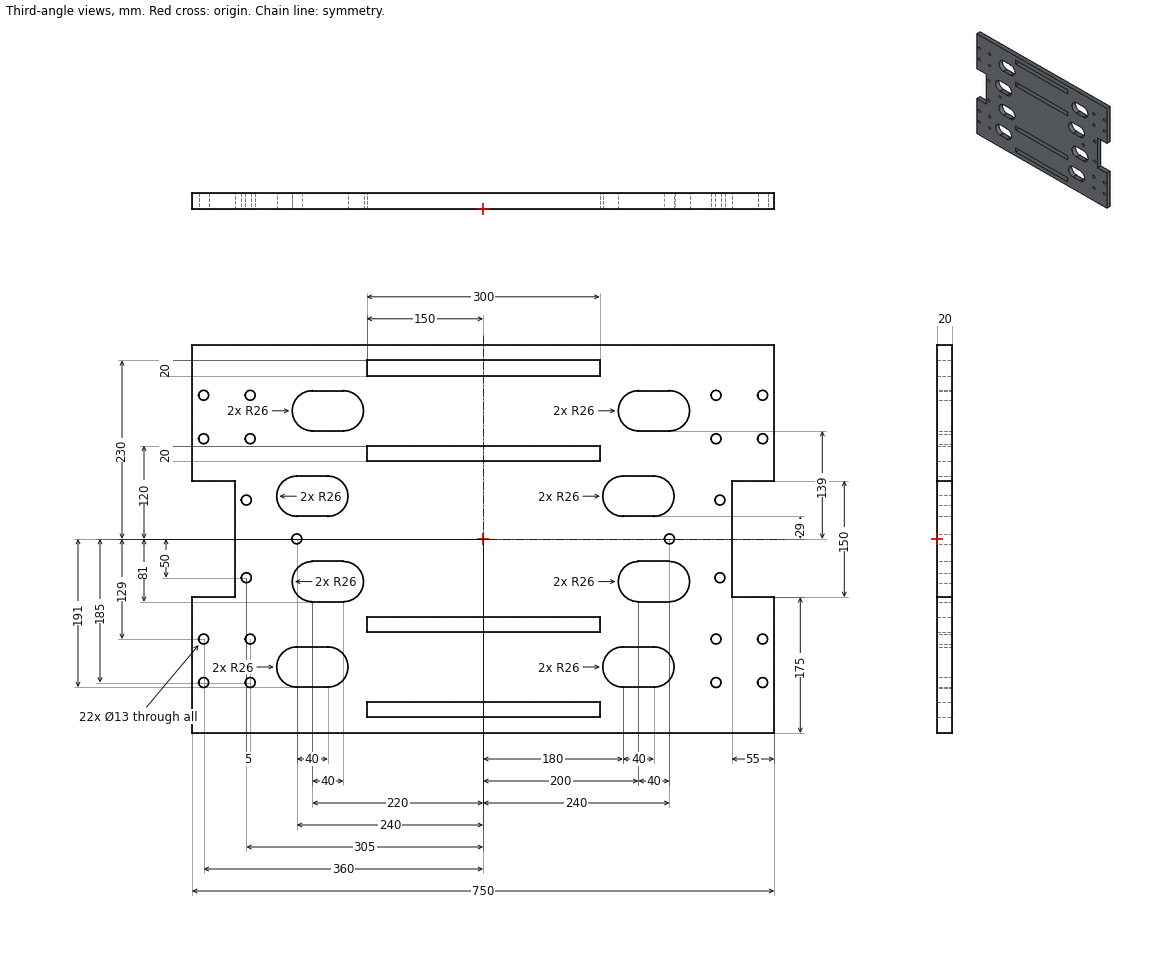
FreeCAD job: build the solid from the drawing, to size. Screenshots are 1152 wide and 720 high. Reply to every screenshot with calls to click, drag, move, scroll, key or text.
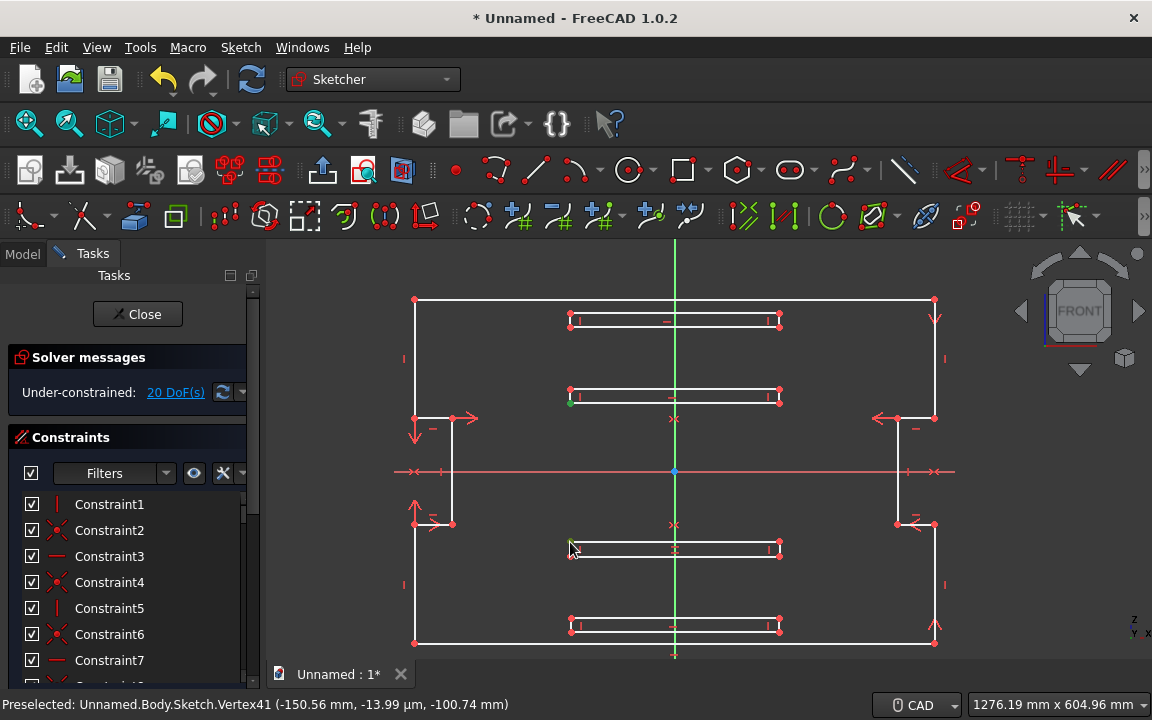
click(393, 472)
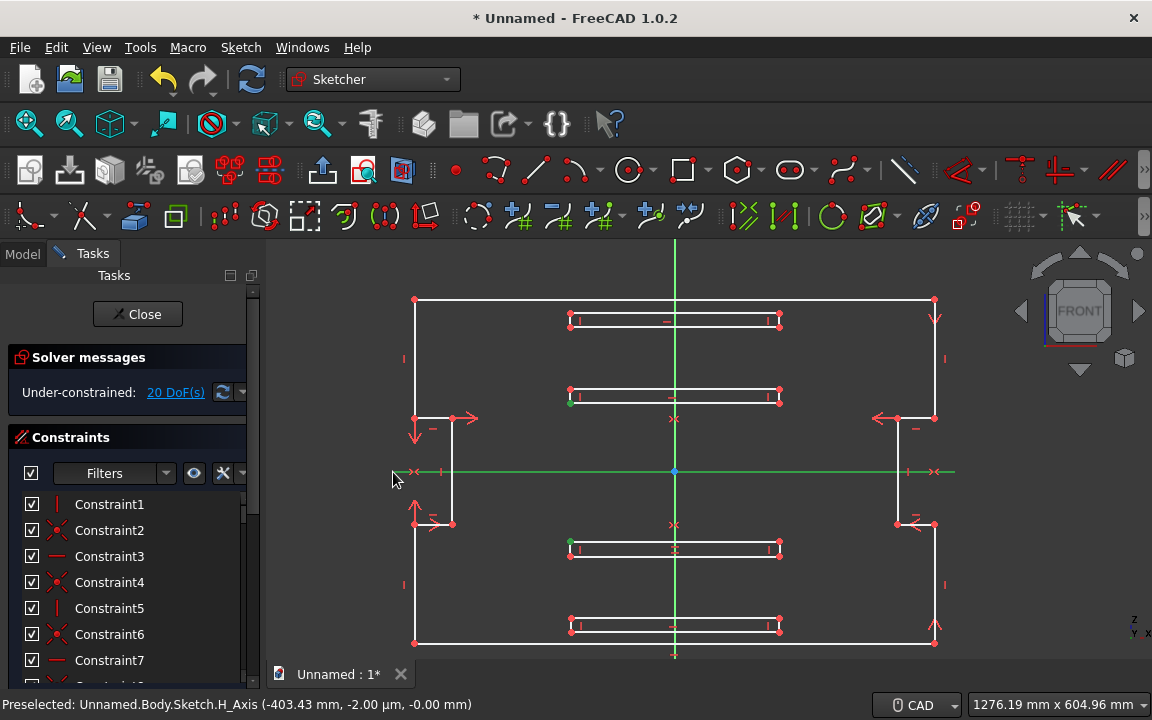
key(s)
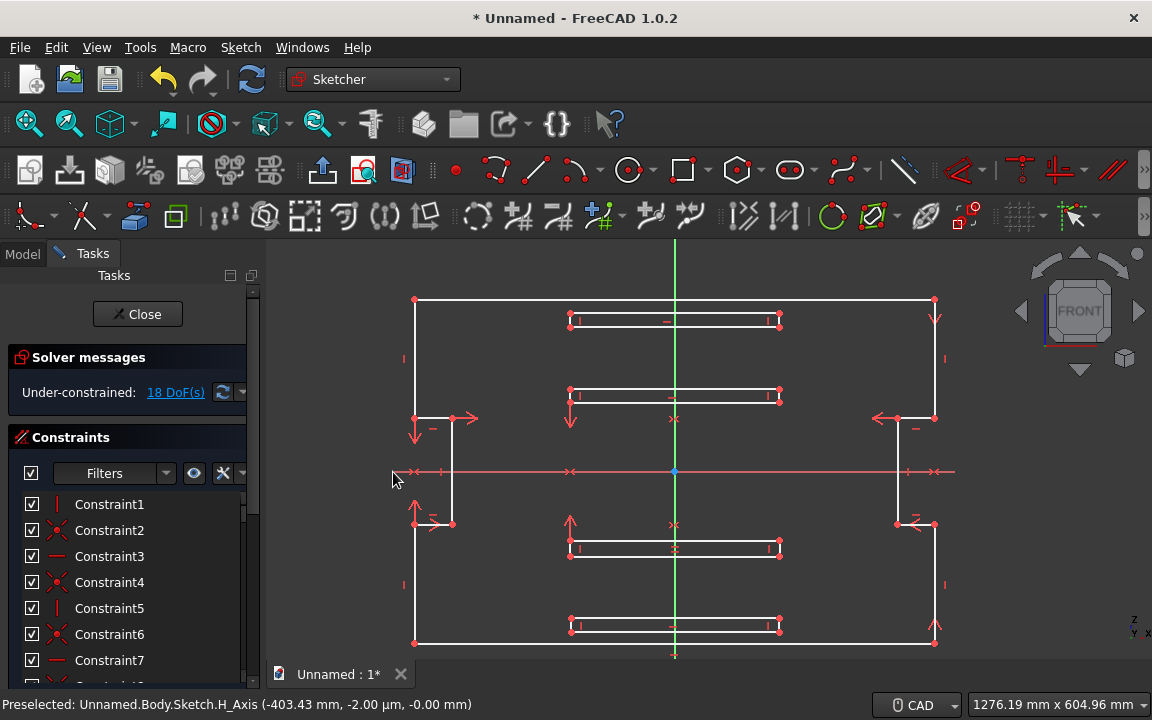
click(779, 389)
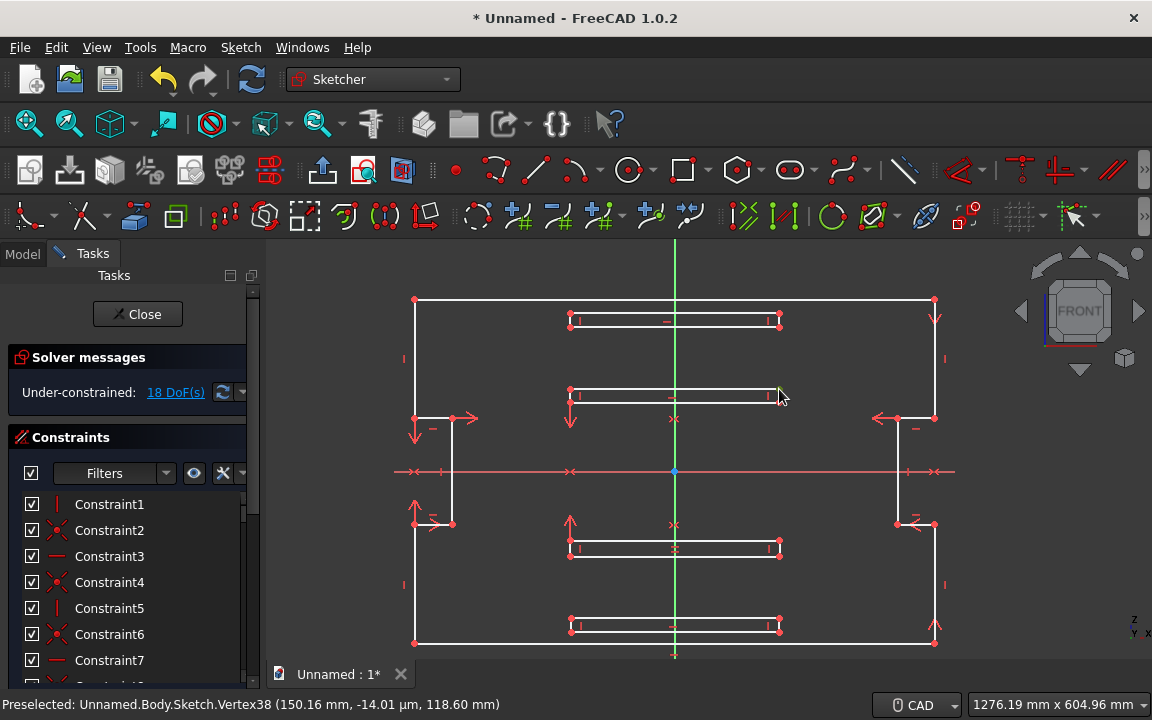
click(780, 557)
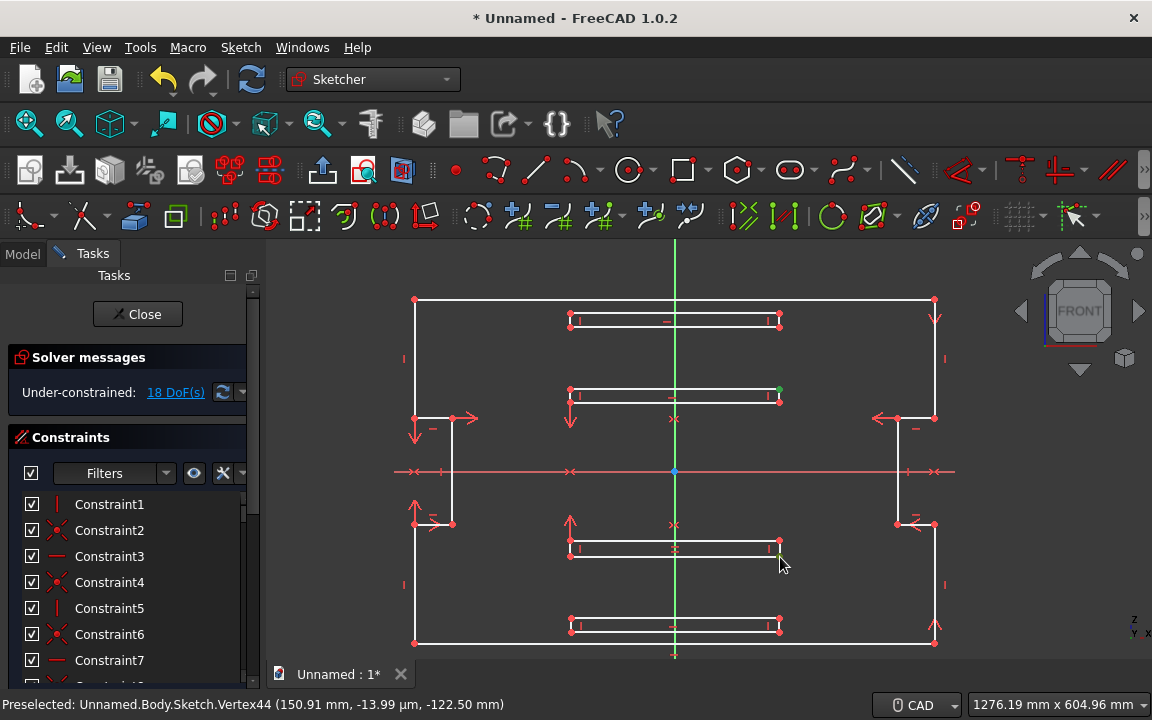
click(393, 472)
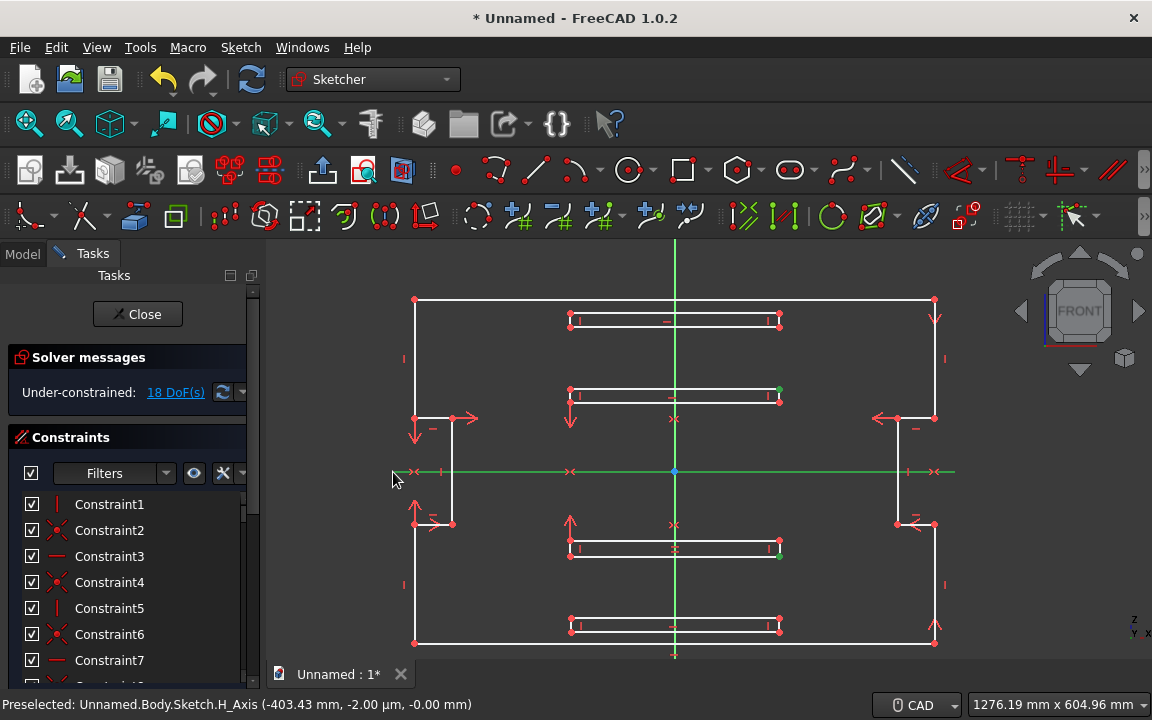
key(s)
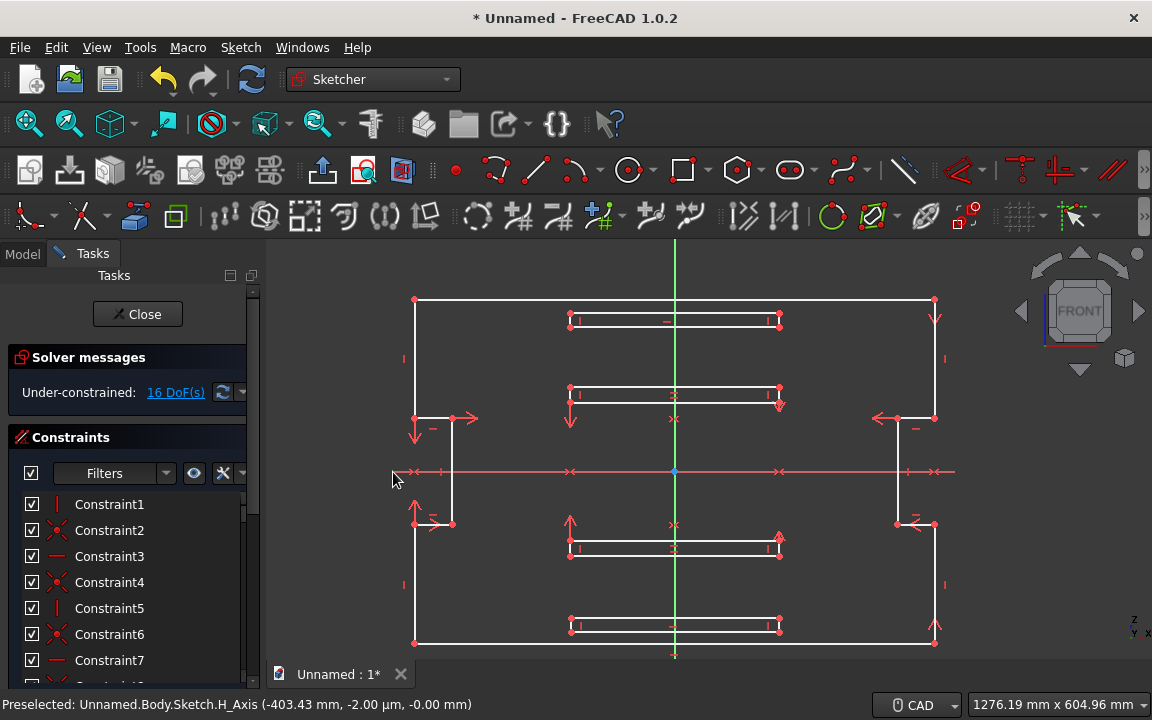
click(570, 327)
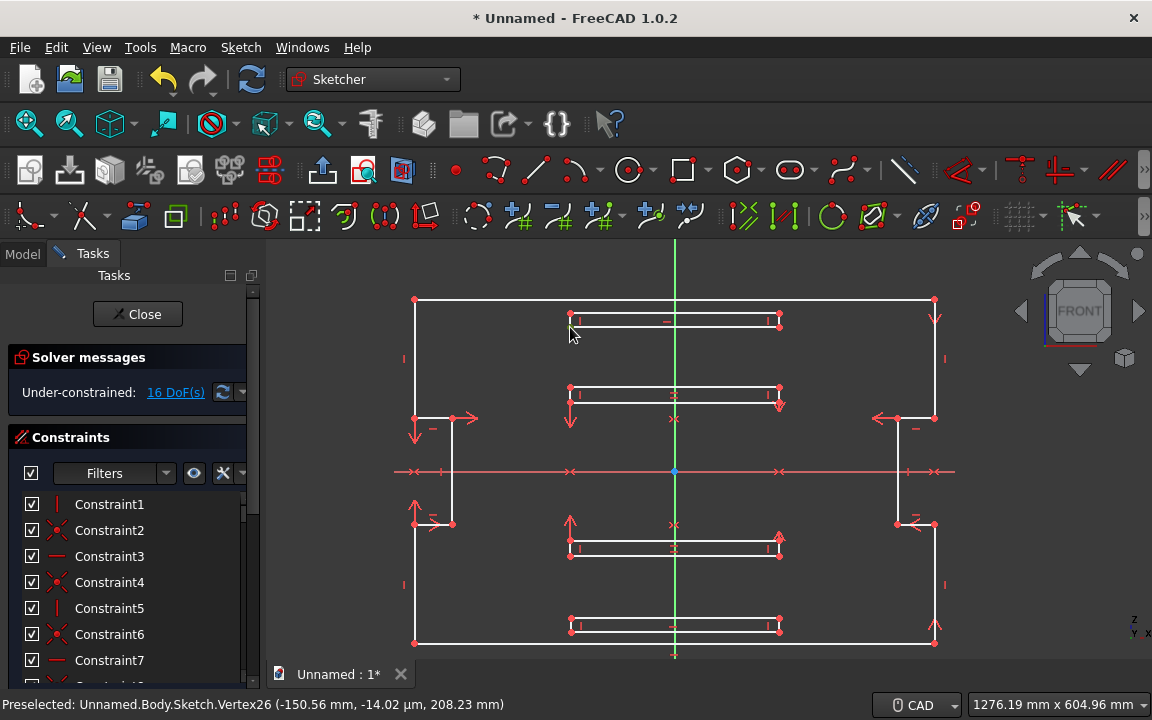
click(571, 618)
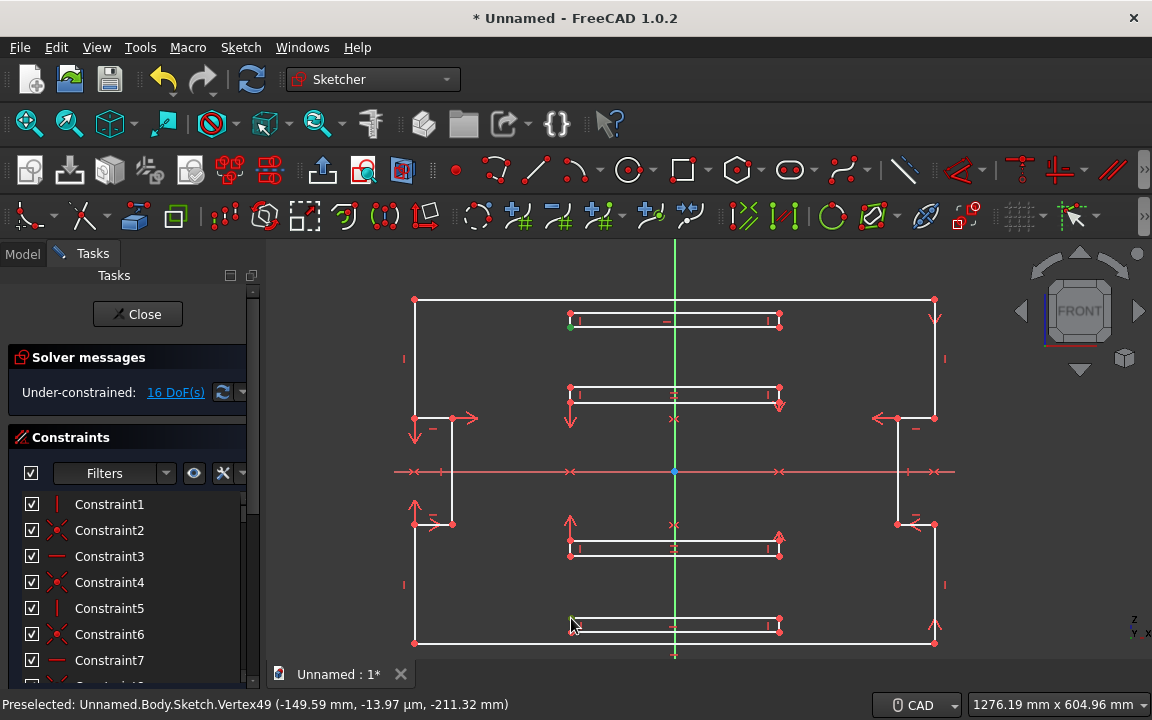
click(393, 472)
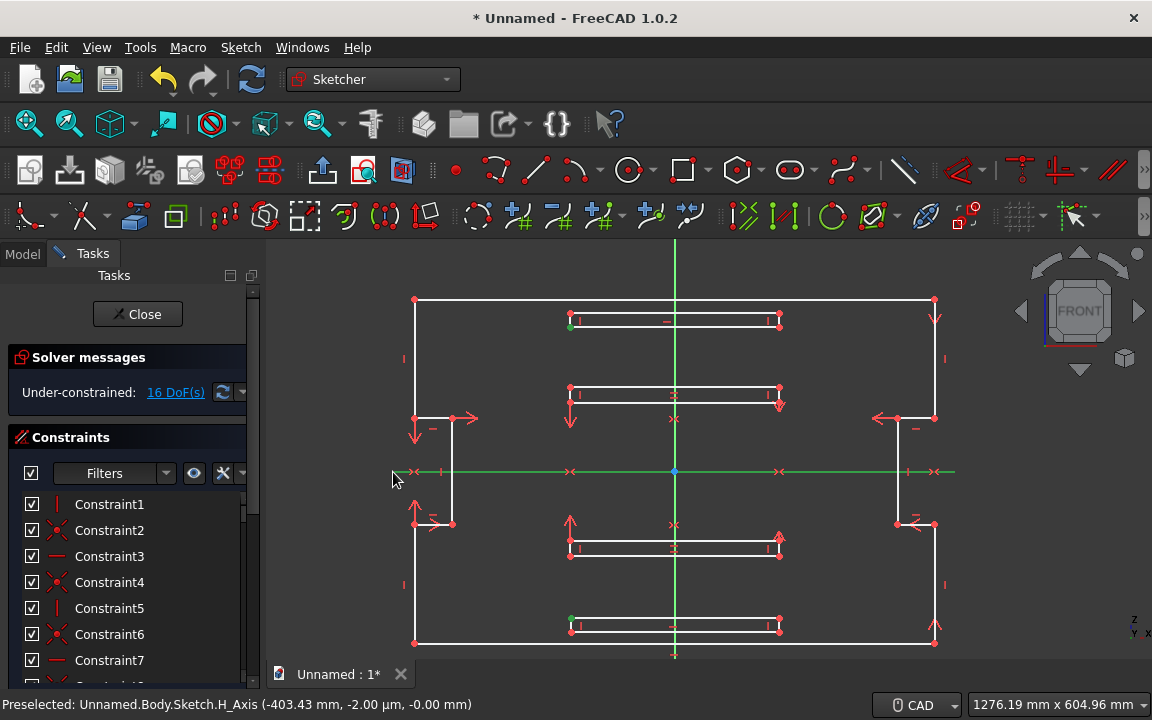
key(s)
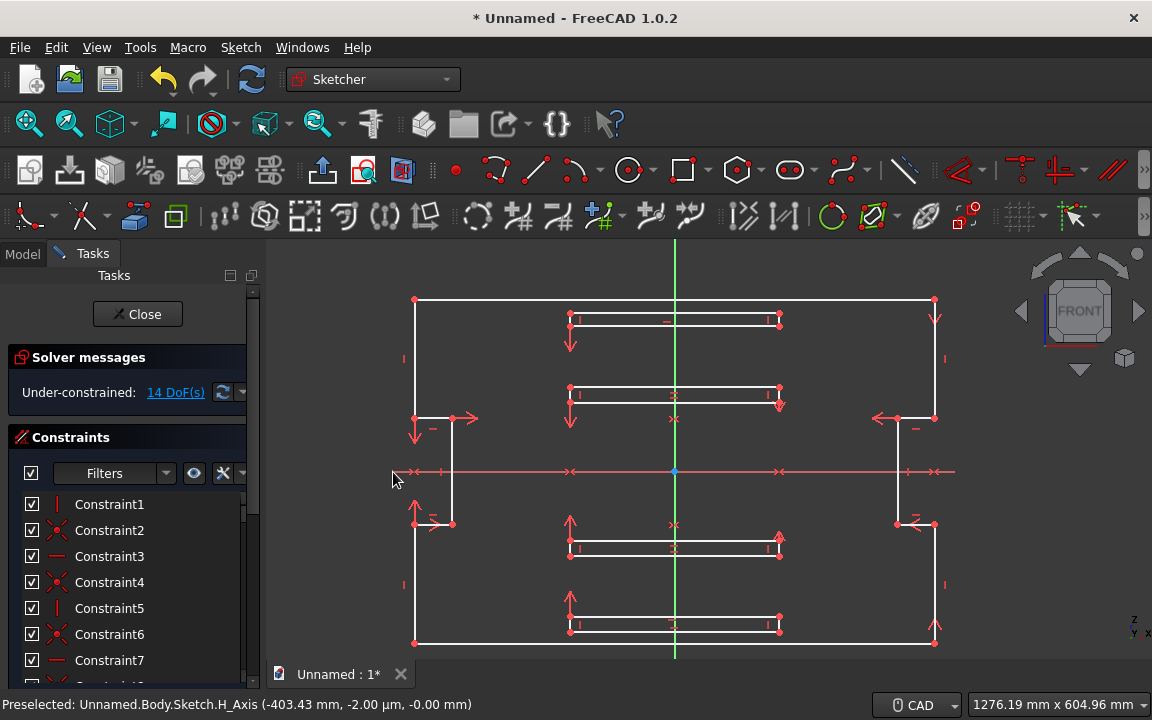
click(779, 313)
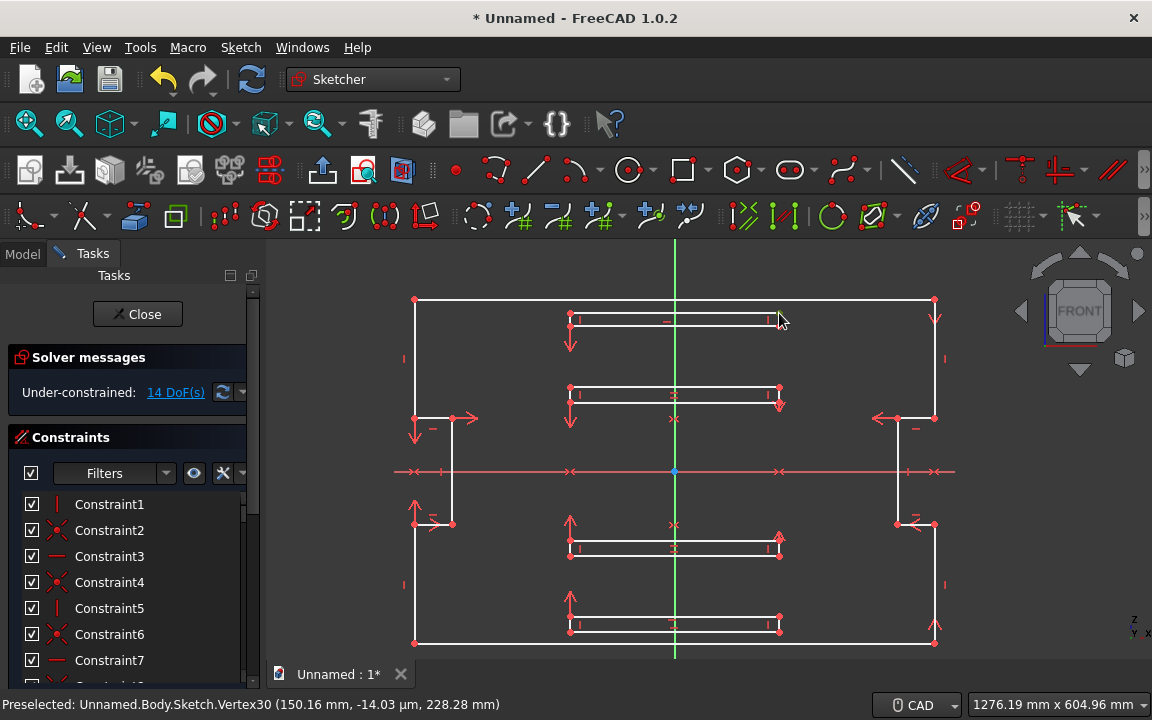
scroll(571, 403, down, 2)